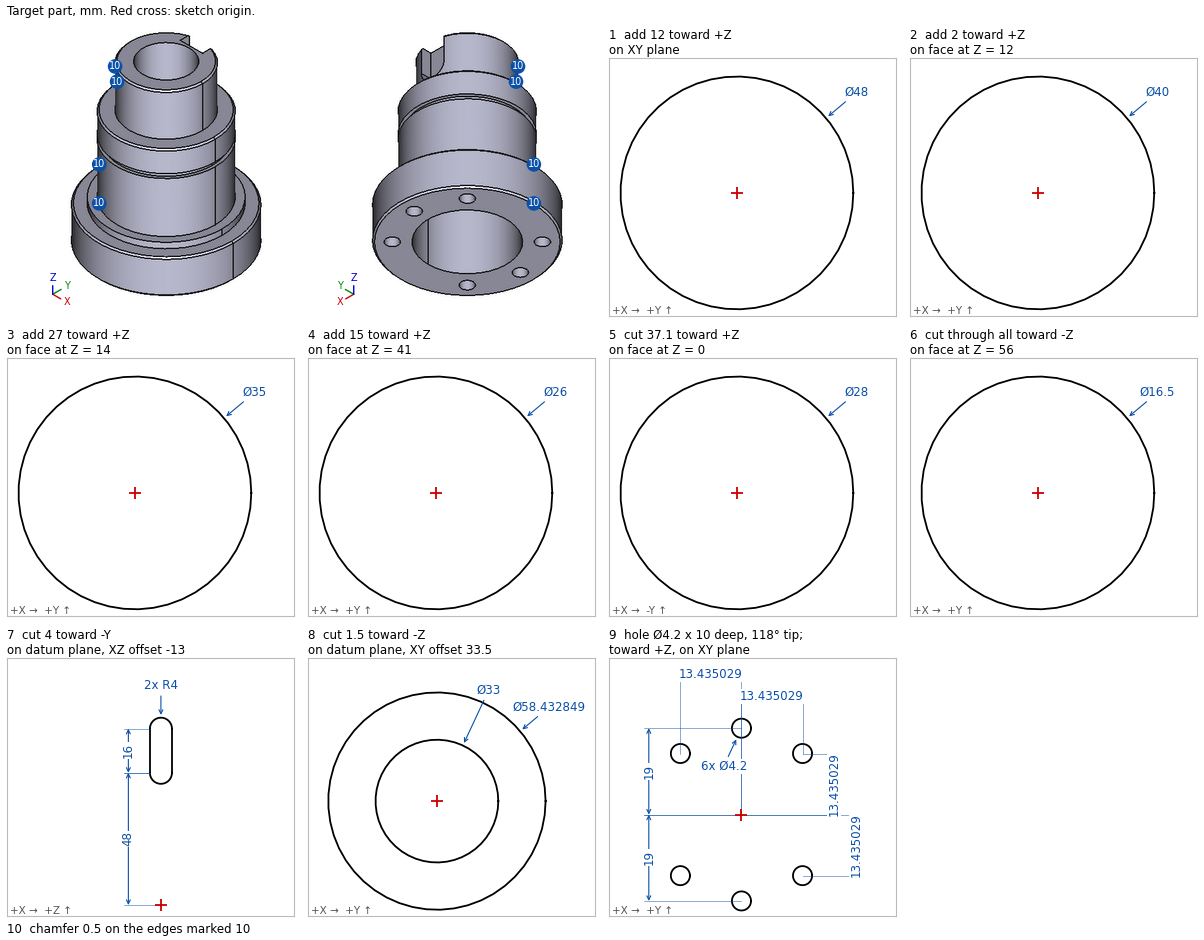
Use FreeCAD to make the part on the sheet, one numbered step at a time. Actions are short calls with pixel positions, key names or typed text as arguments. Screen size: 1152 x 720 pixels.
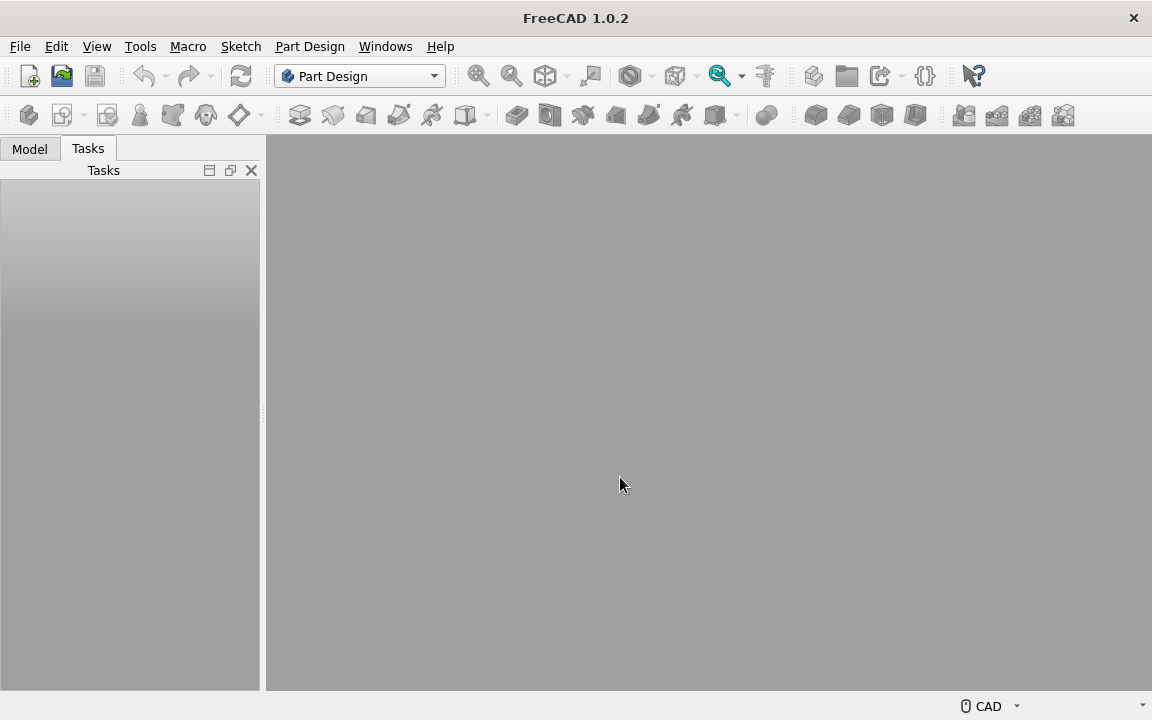
key(ctrl+n)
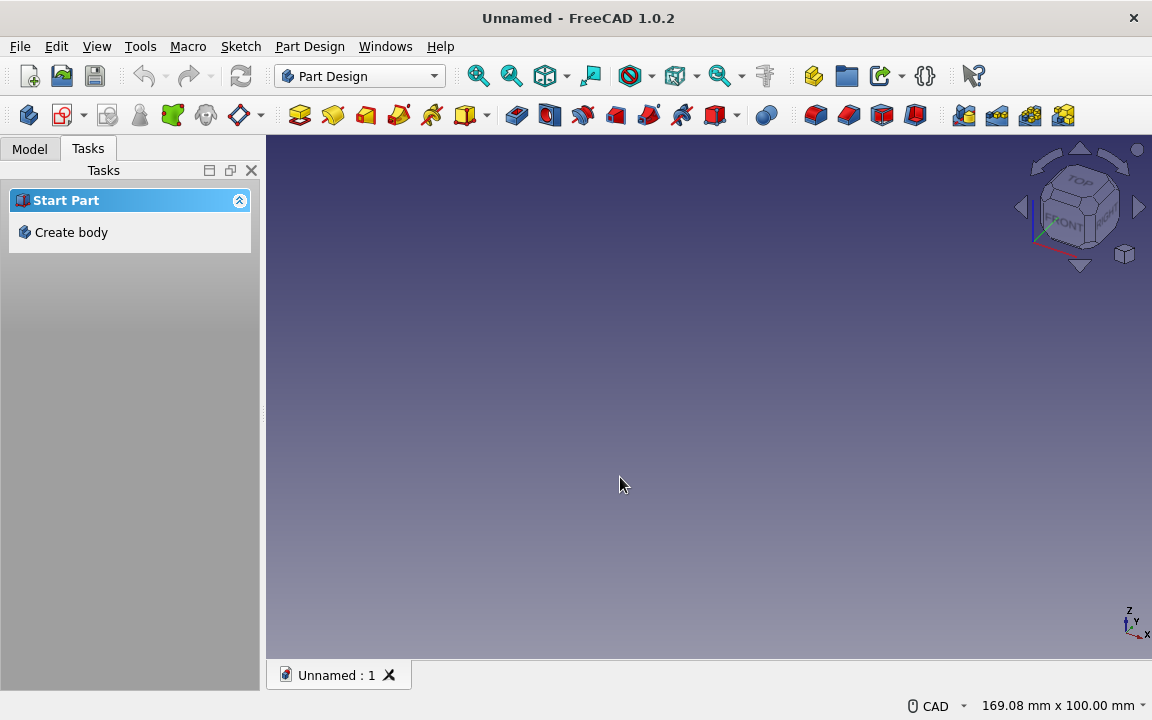
click(62, 116)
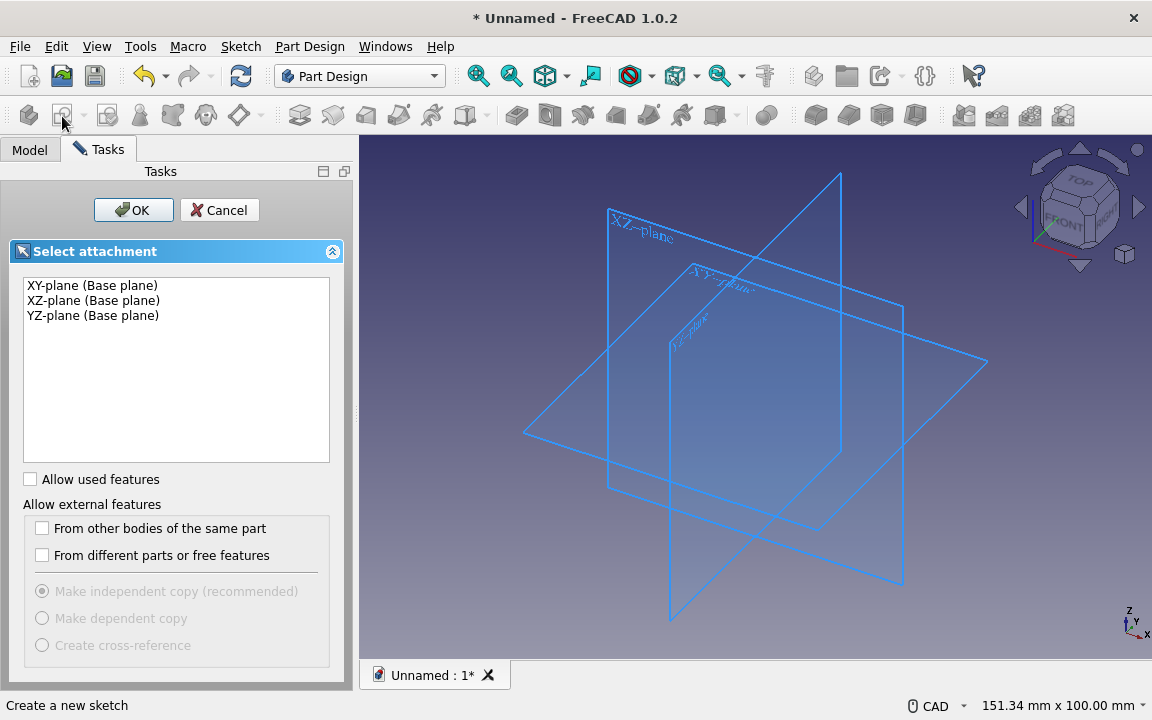
click(84, 286)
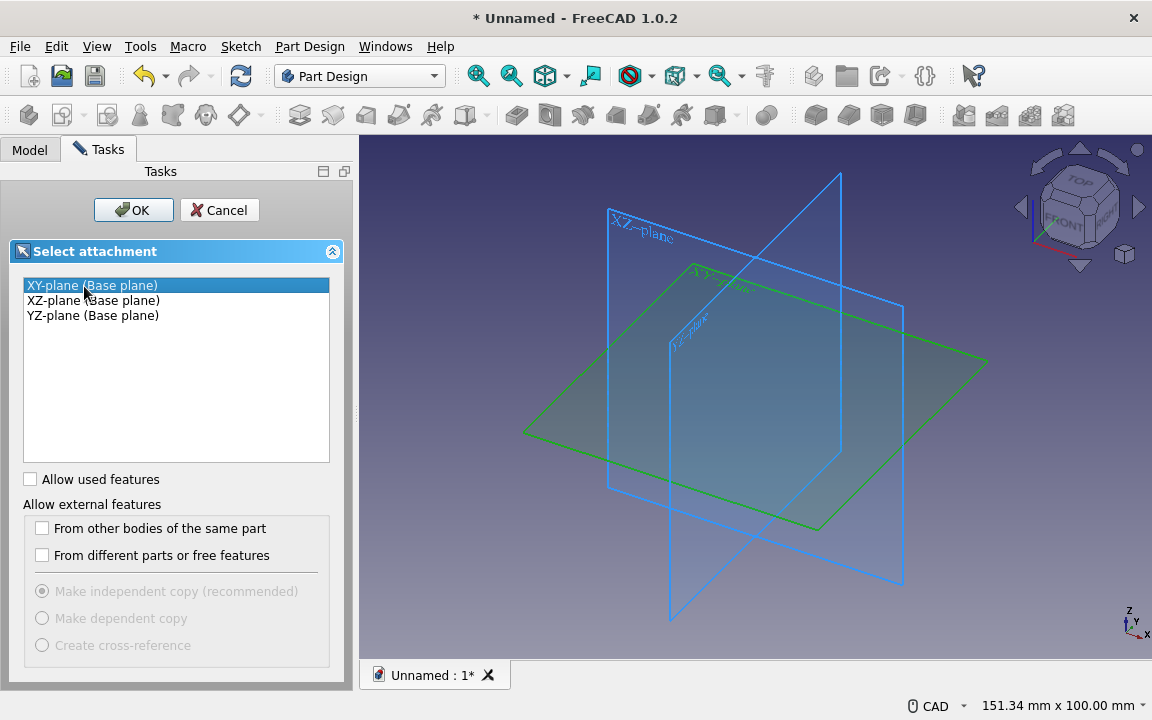
click(134, 210)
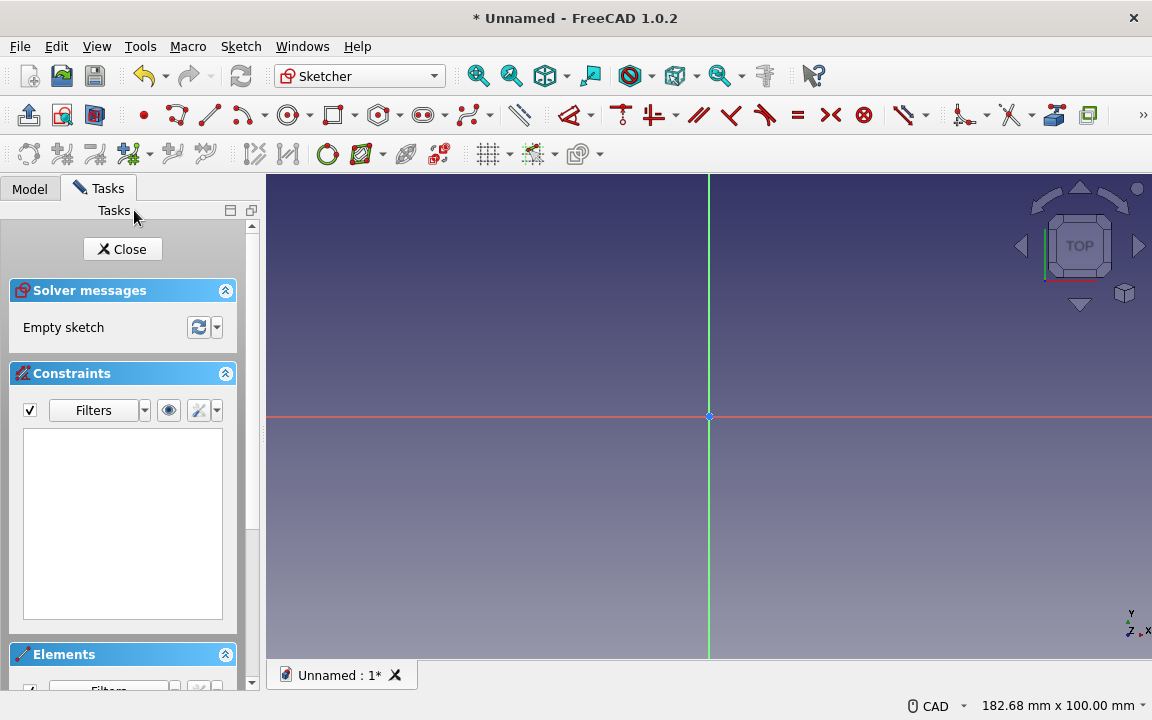
key(g)
key(c)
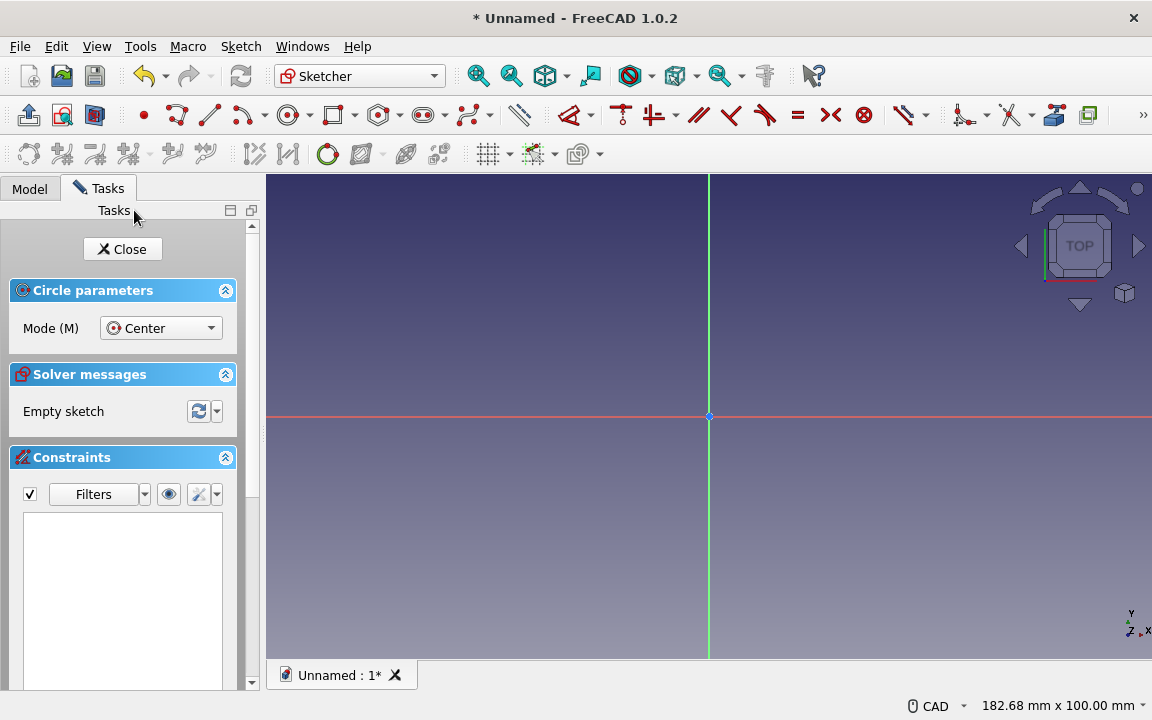
click(709, 416)
click(791, 334)
key(Escape)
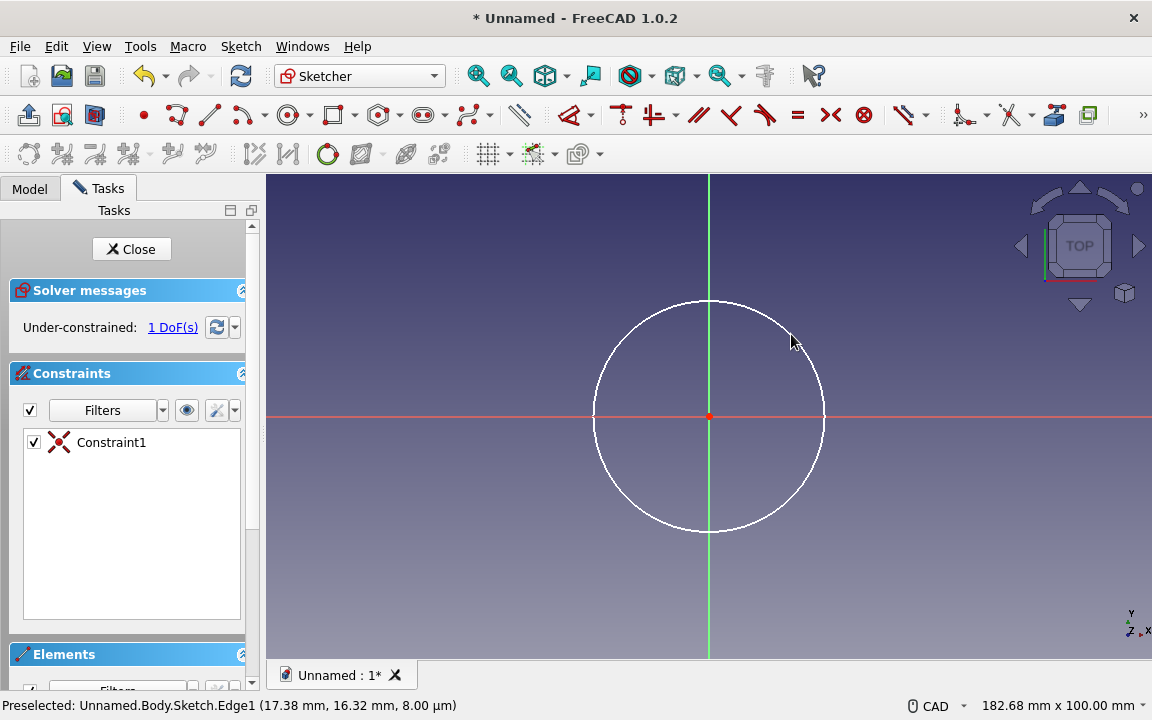
click(790, 334)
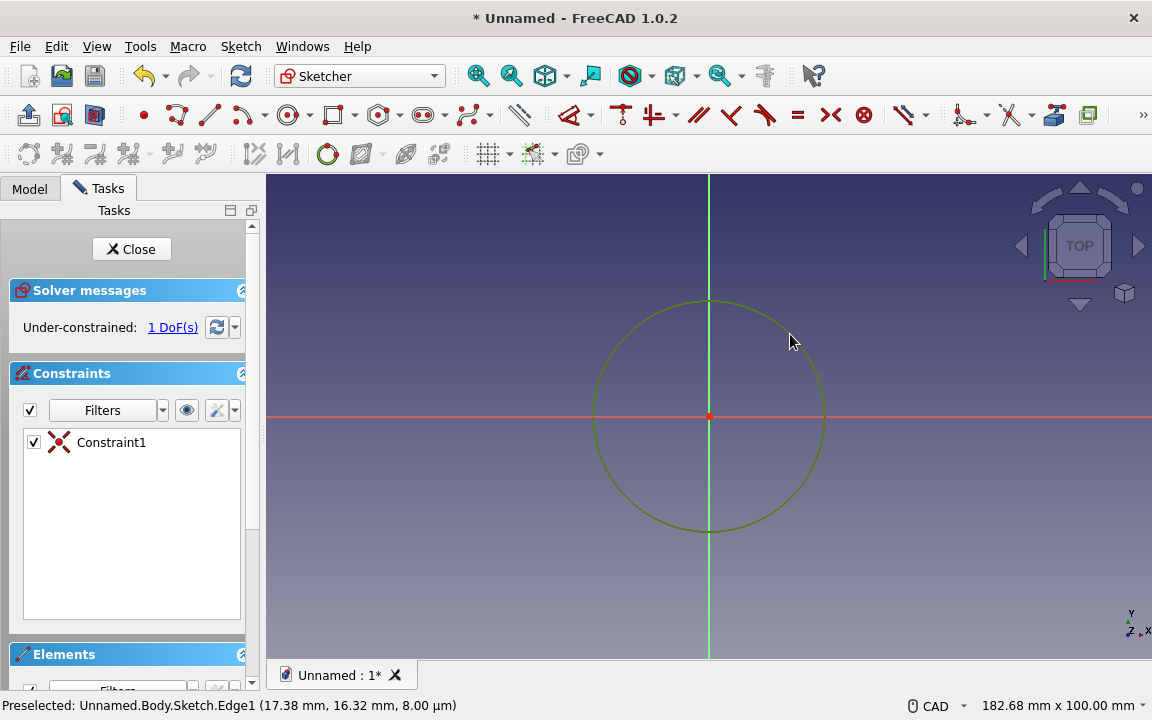
key(k)
key(o)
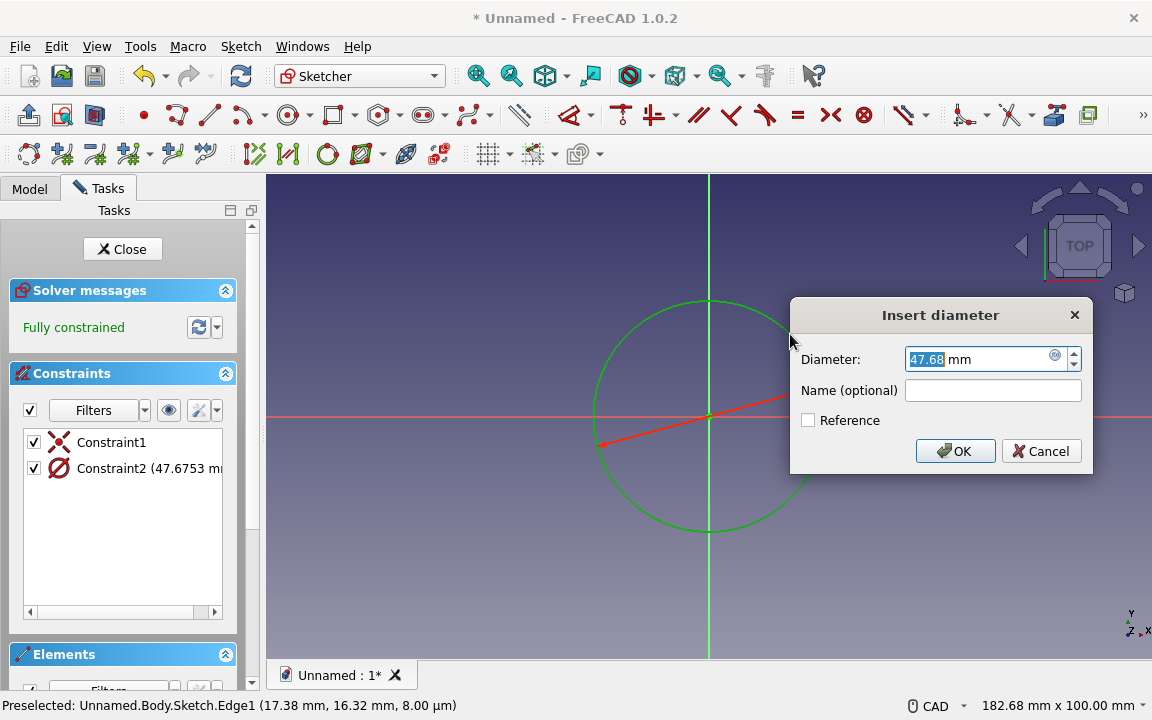
text(48)
key(Return)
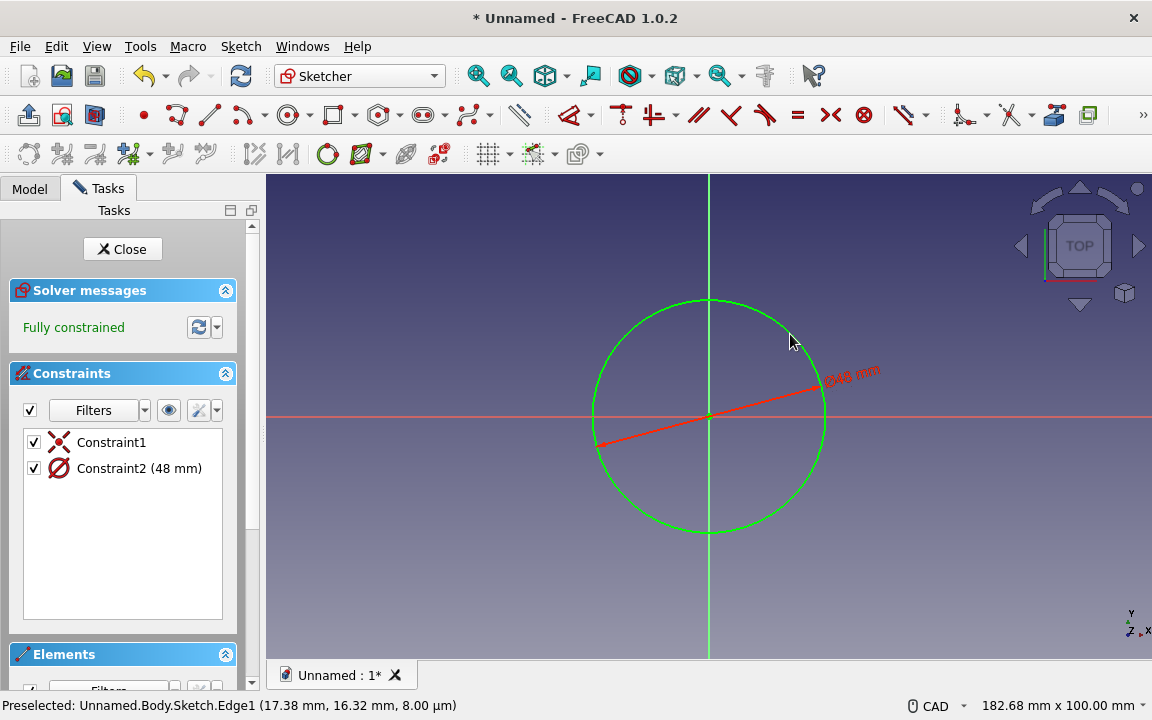
click(123, 249)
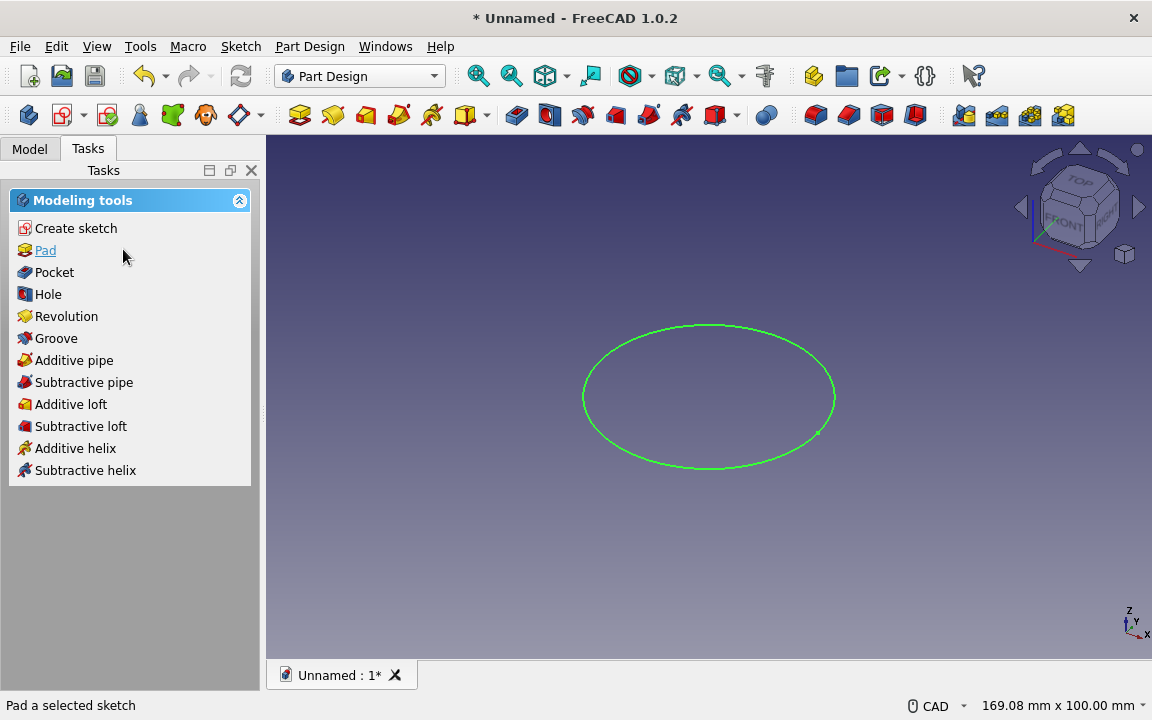
click(300, 116)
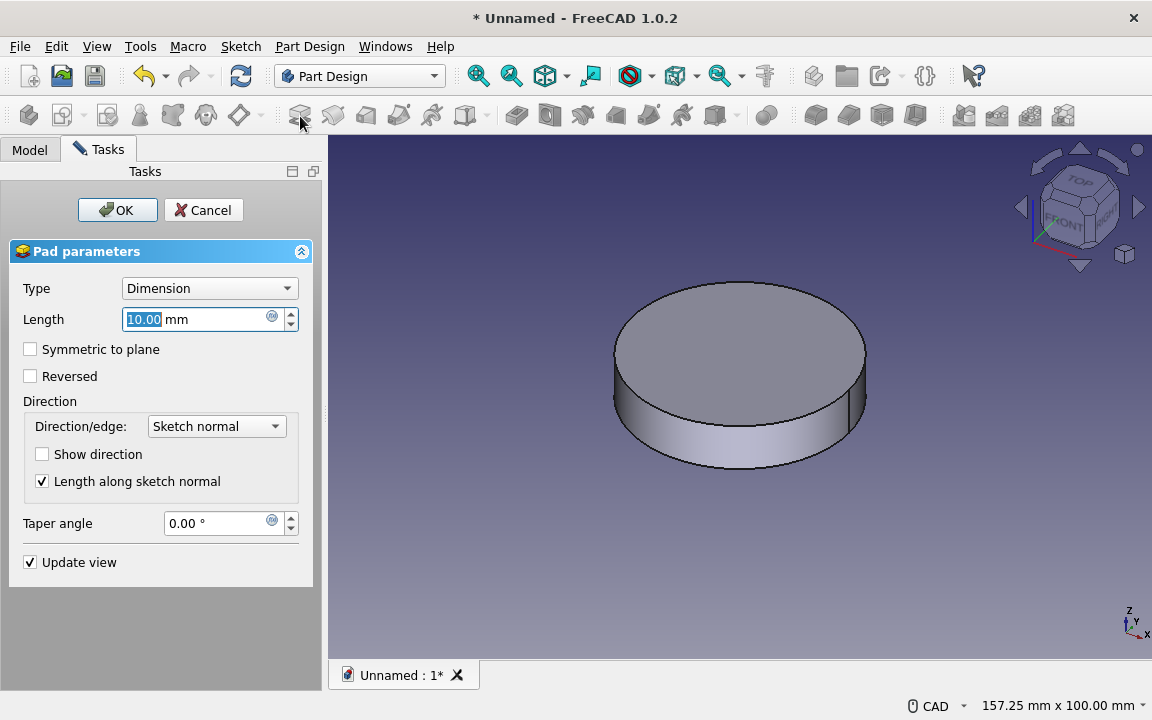
text(12)
key(Tab)